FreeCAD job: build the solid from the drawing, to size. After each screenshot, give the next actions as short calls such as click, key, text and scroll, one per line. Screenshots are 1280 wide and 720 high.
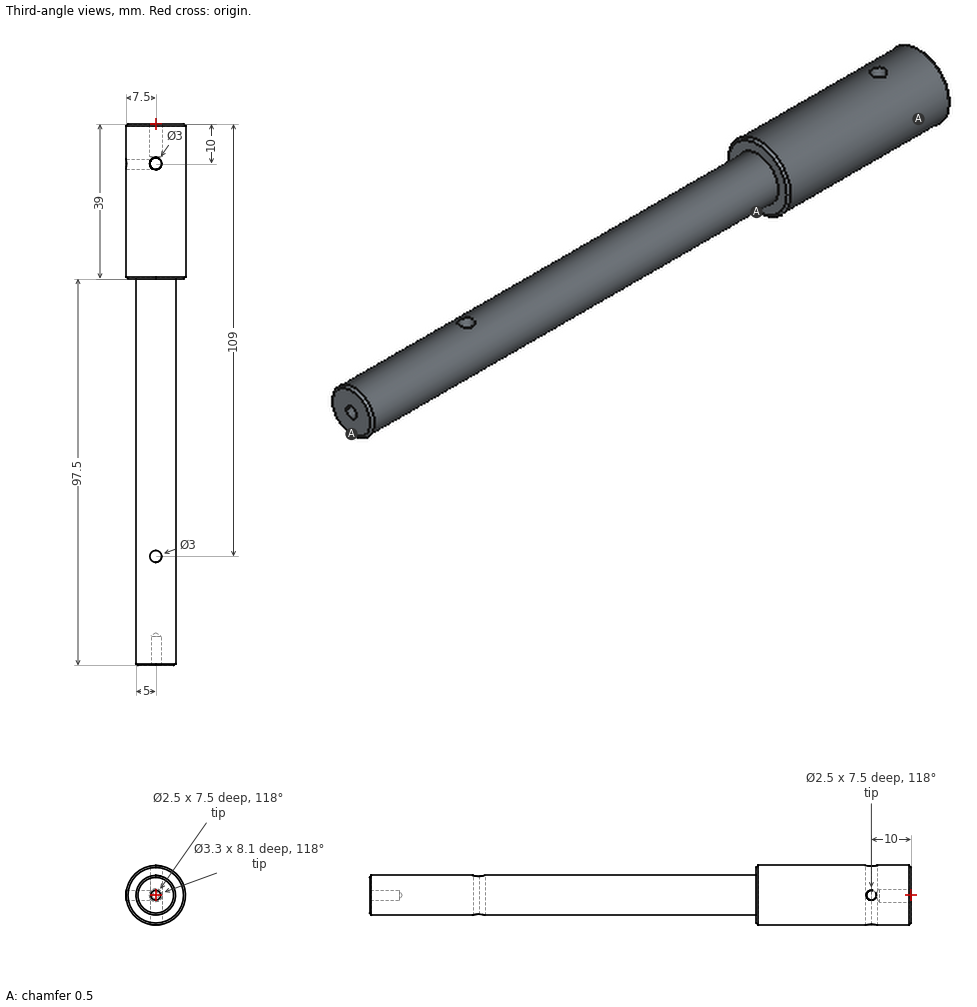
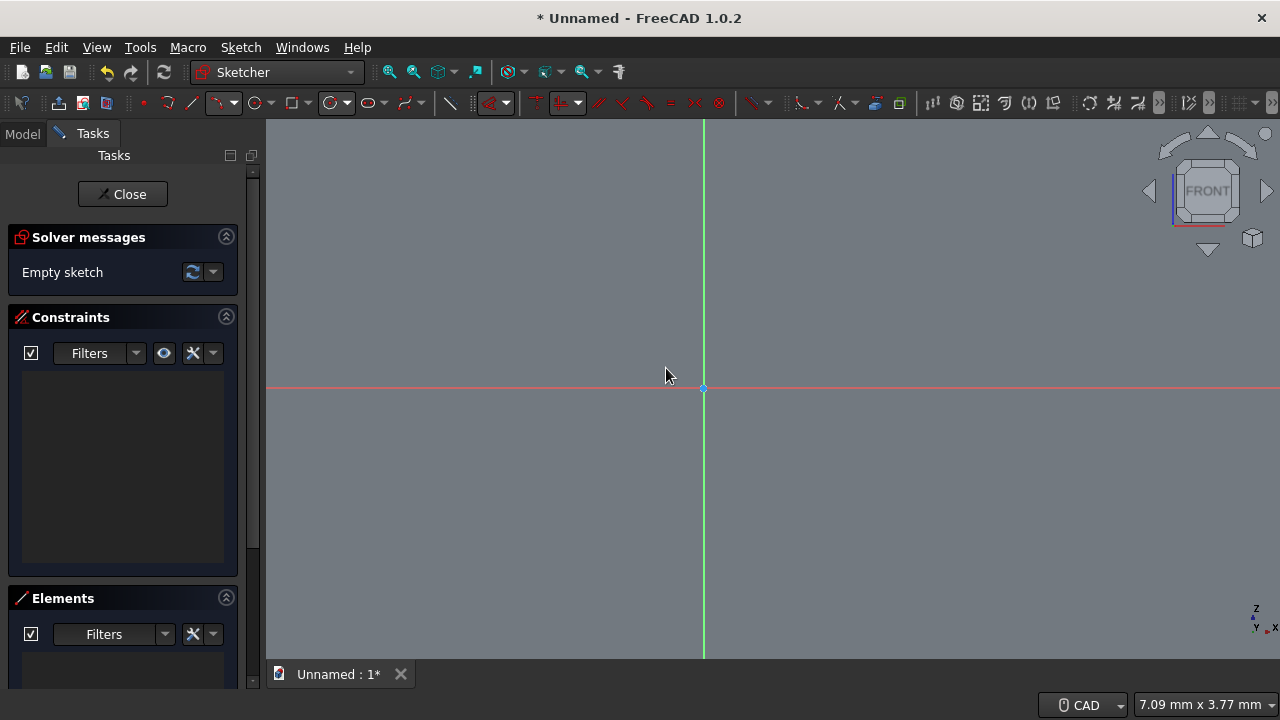
click(256, 104)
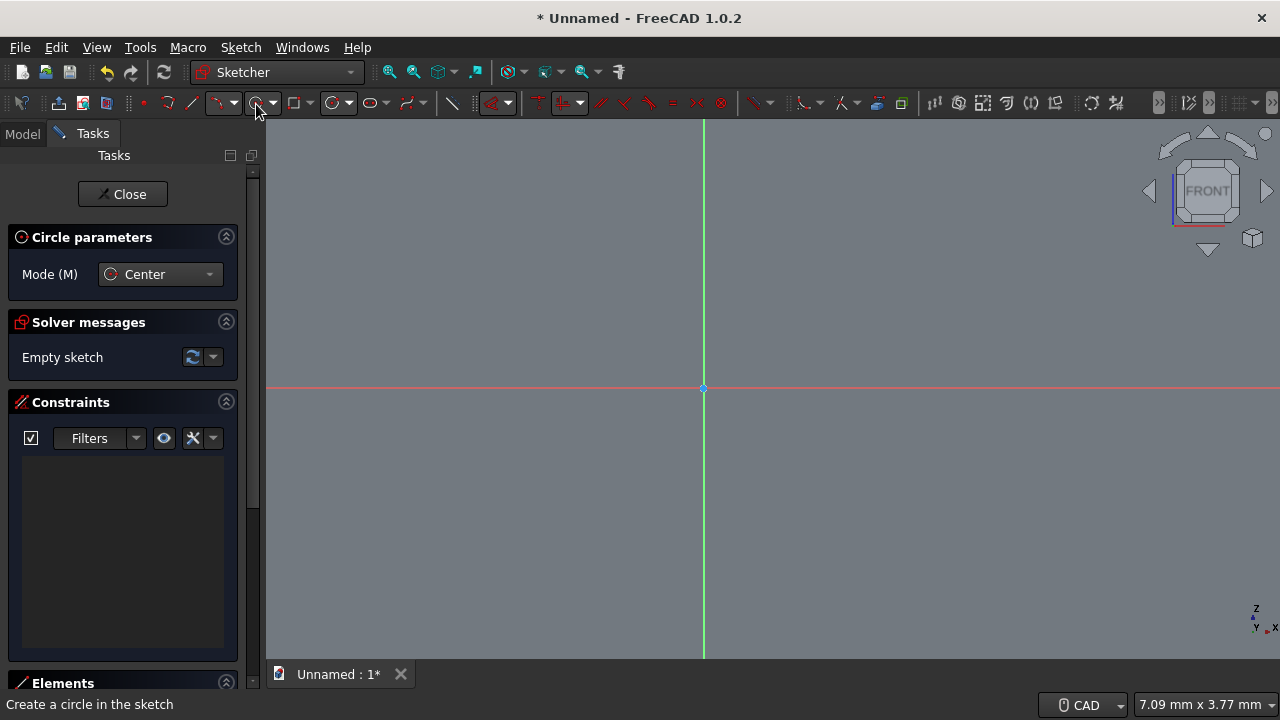
click(704, 388)
click(830, 262)
key(Escape)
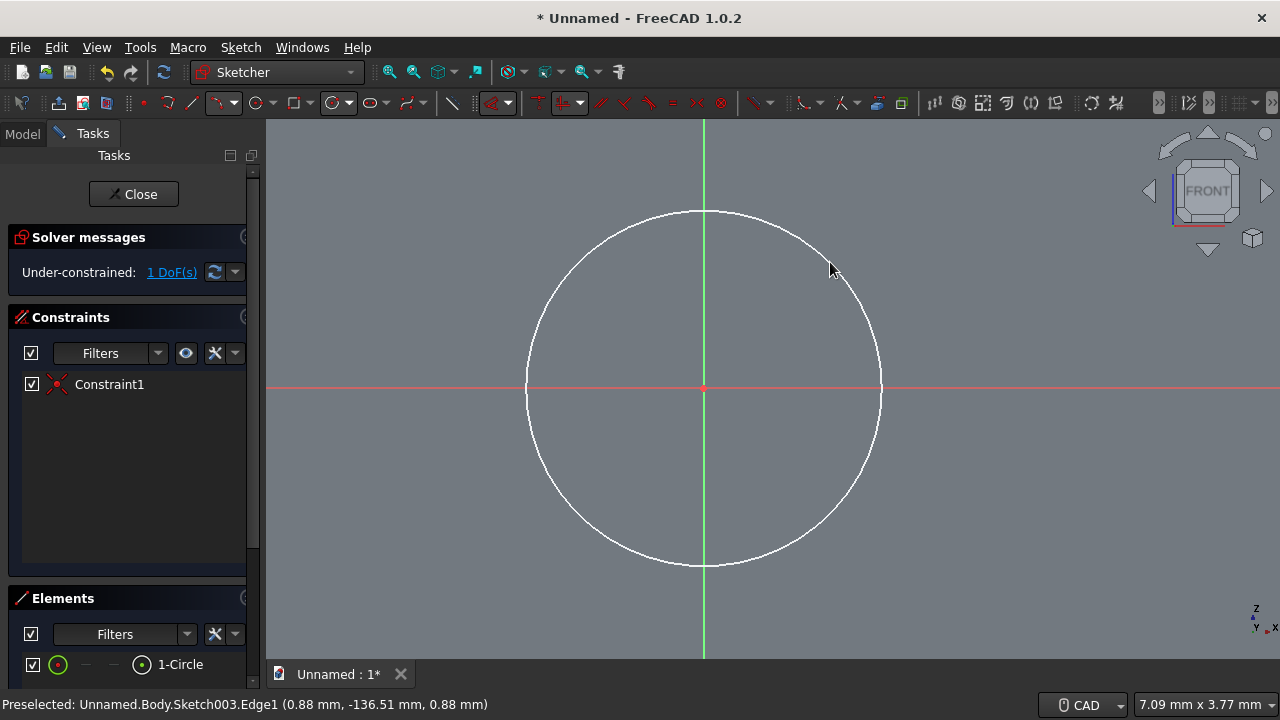
click(829, 262)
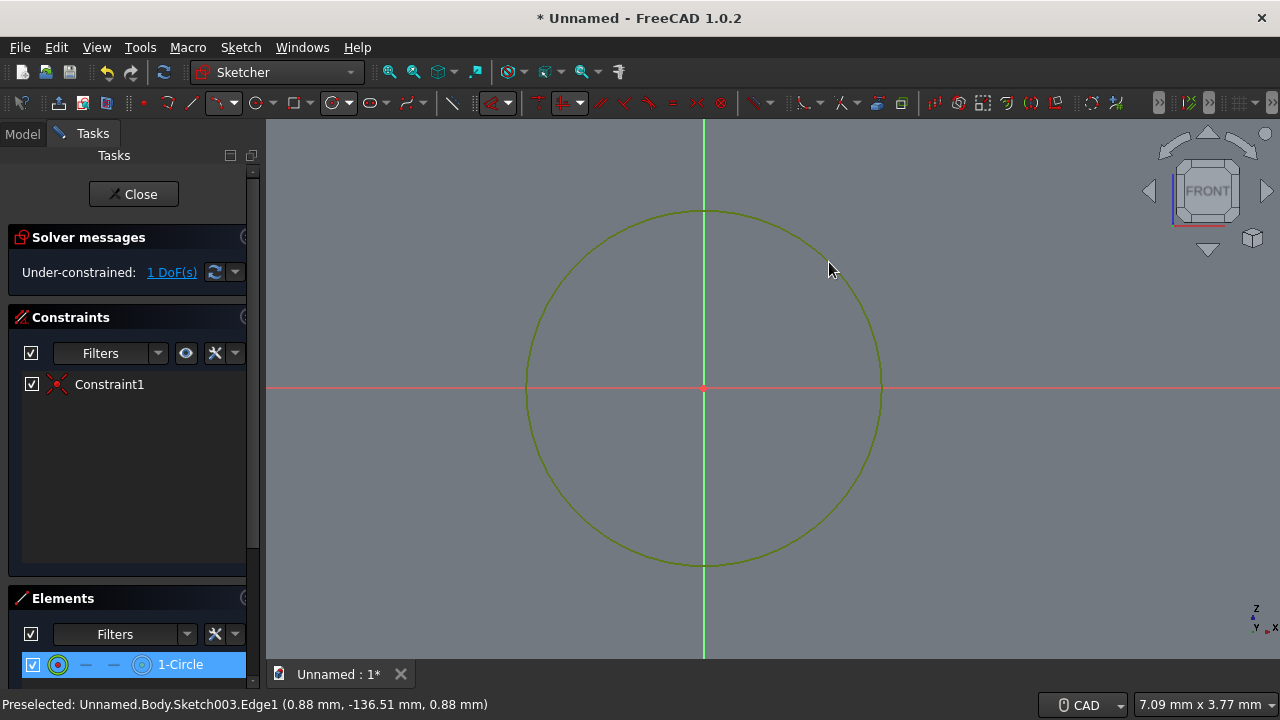
click(510, 104)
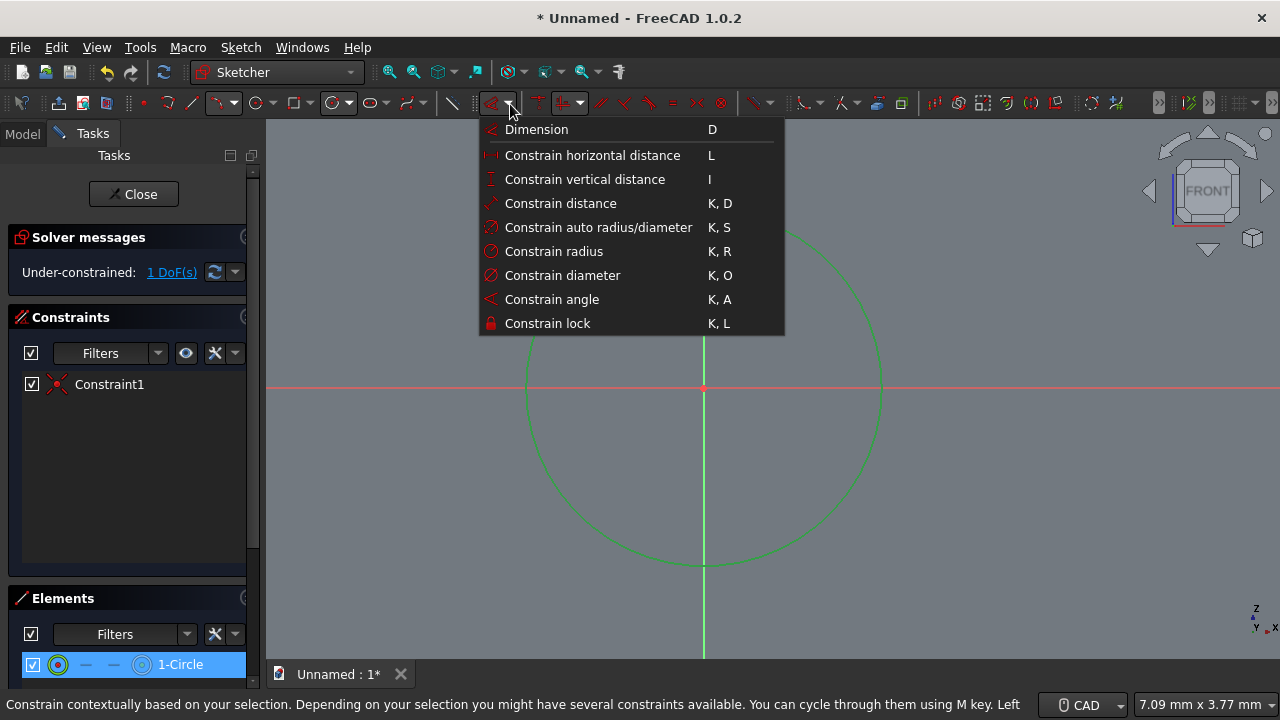
click(632, 275)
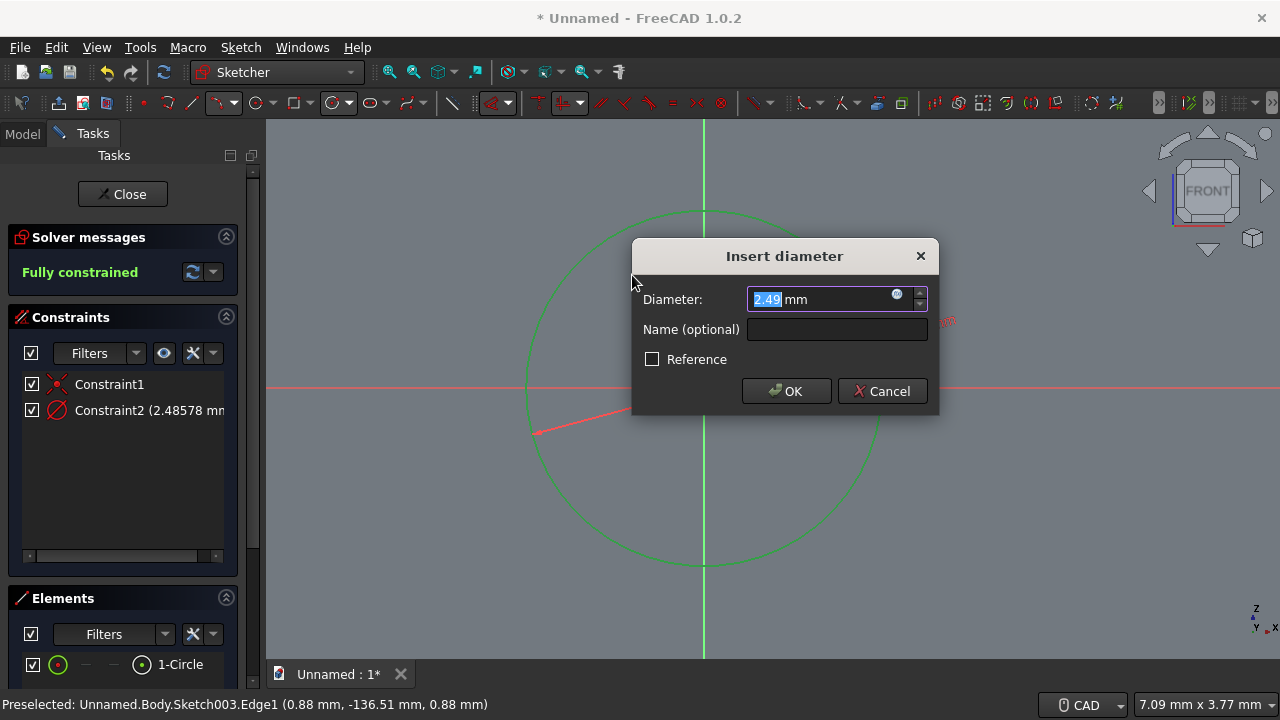
text(2.5)
key(Return)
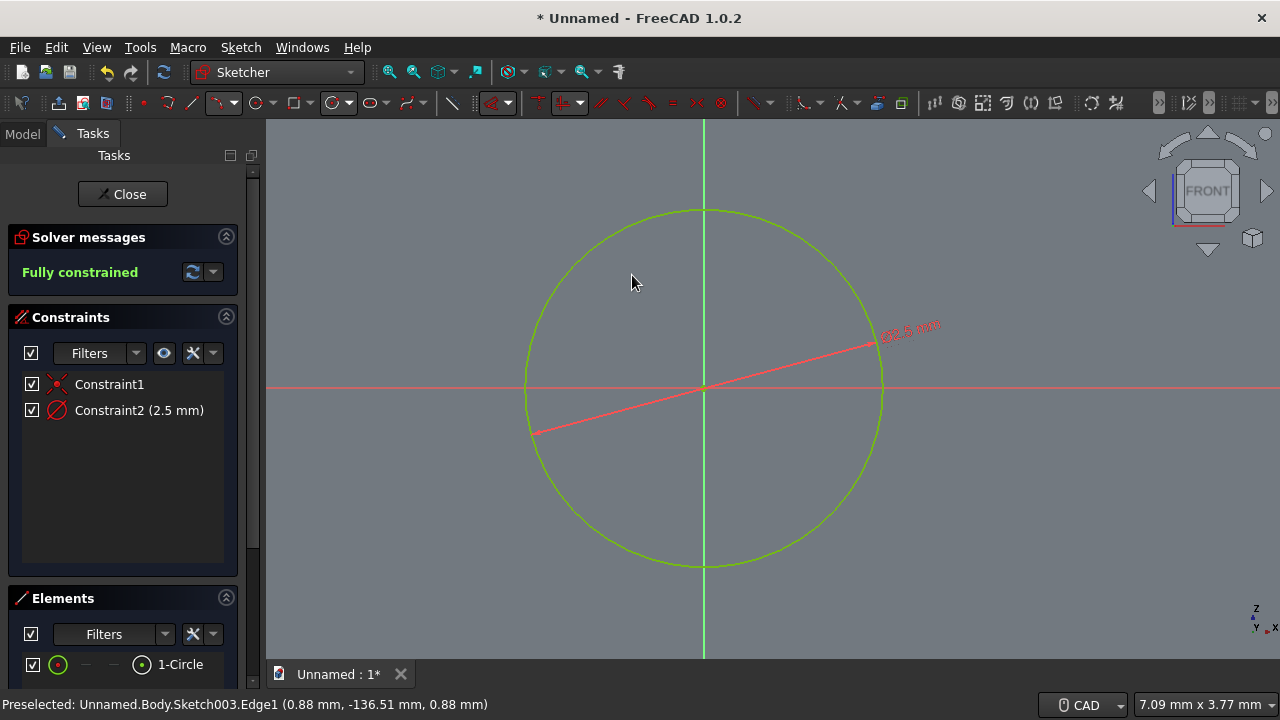
click(123, 194)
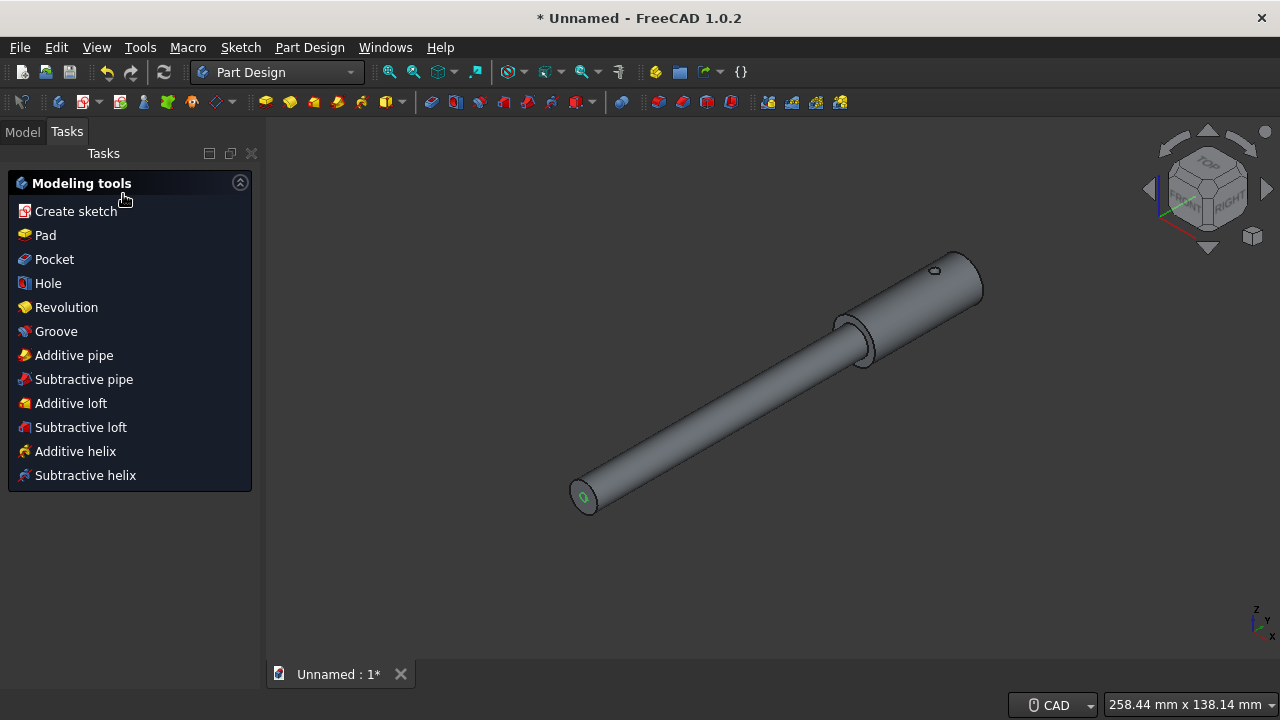
click(456, 102)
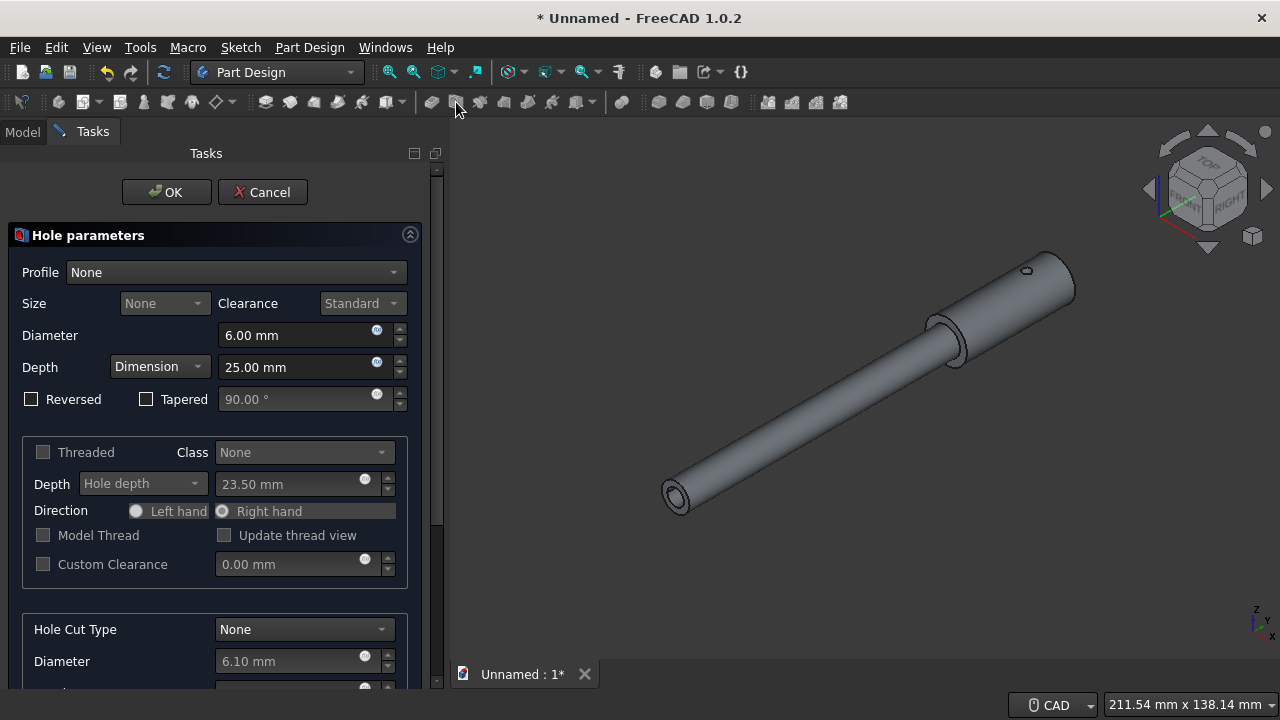
triple_click(305, 335)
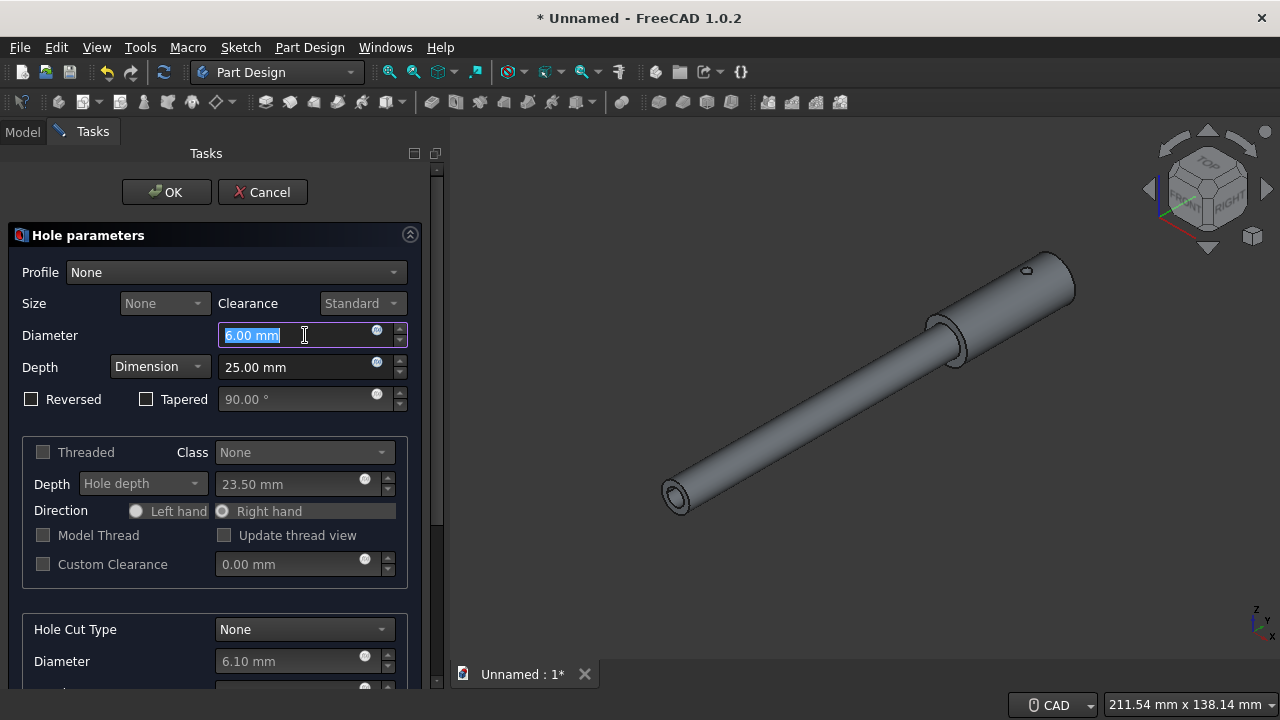
text(2.5)
key(Tab)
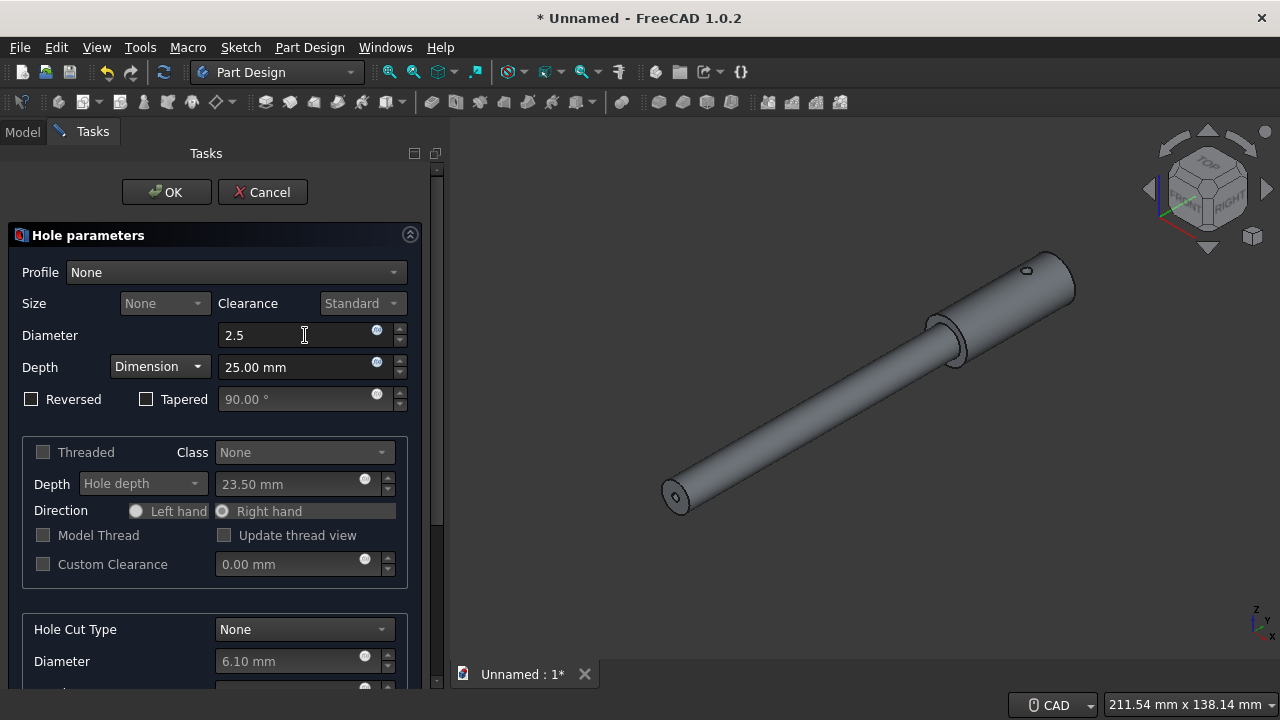
triple_click(305, 367)